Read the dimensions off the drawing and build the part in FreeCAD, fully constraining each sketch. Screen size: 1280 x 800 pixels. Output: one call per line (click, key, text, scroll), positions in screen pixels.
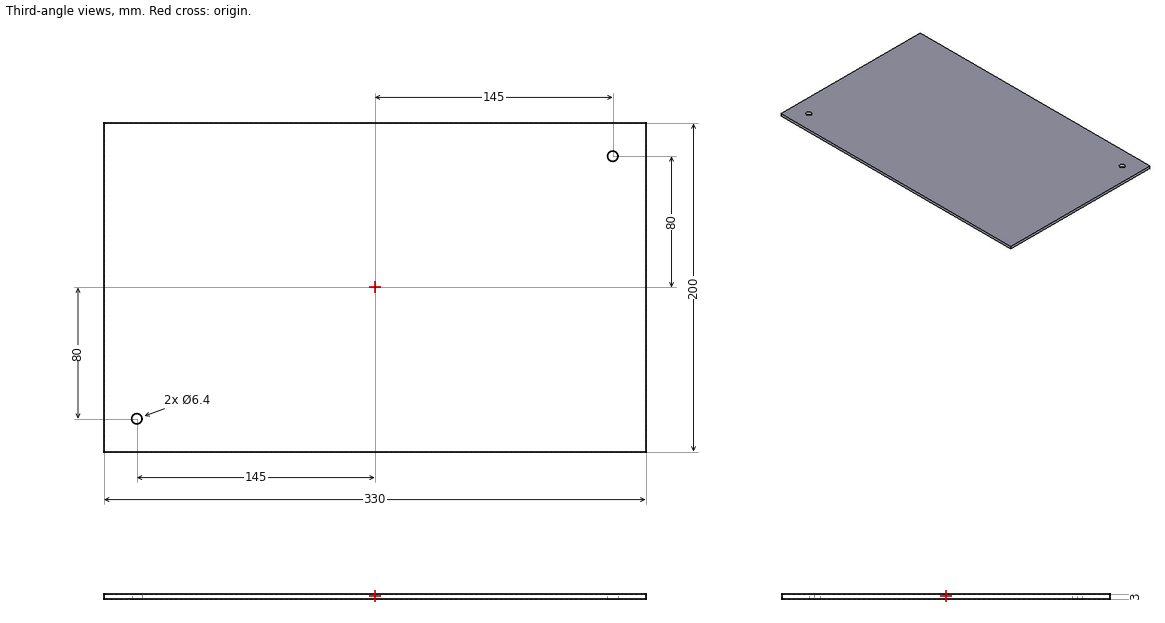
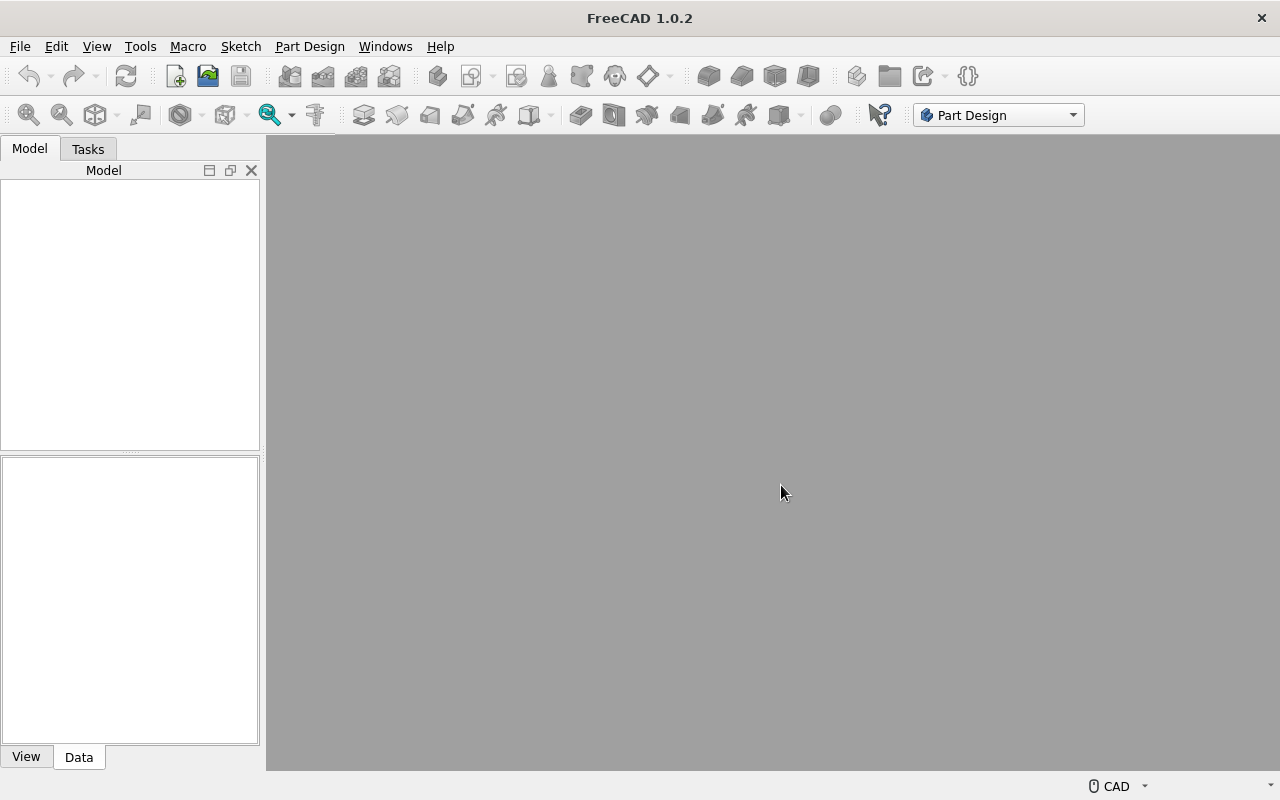
click(175, 76)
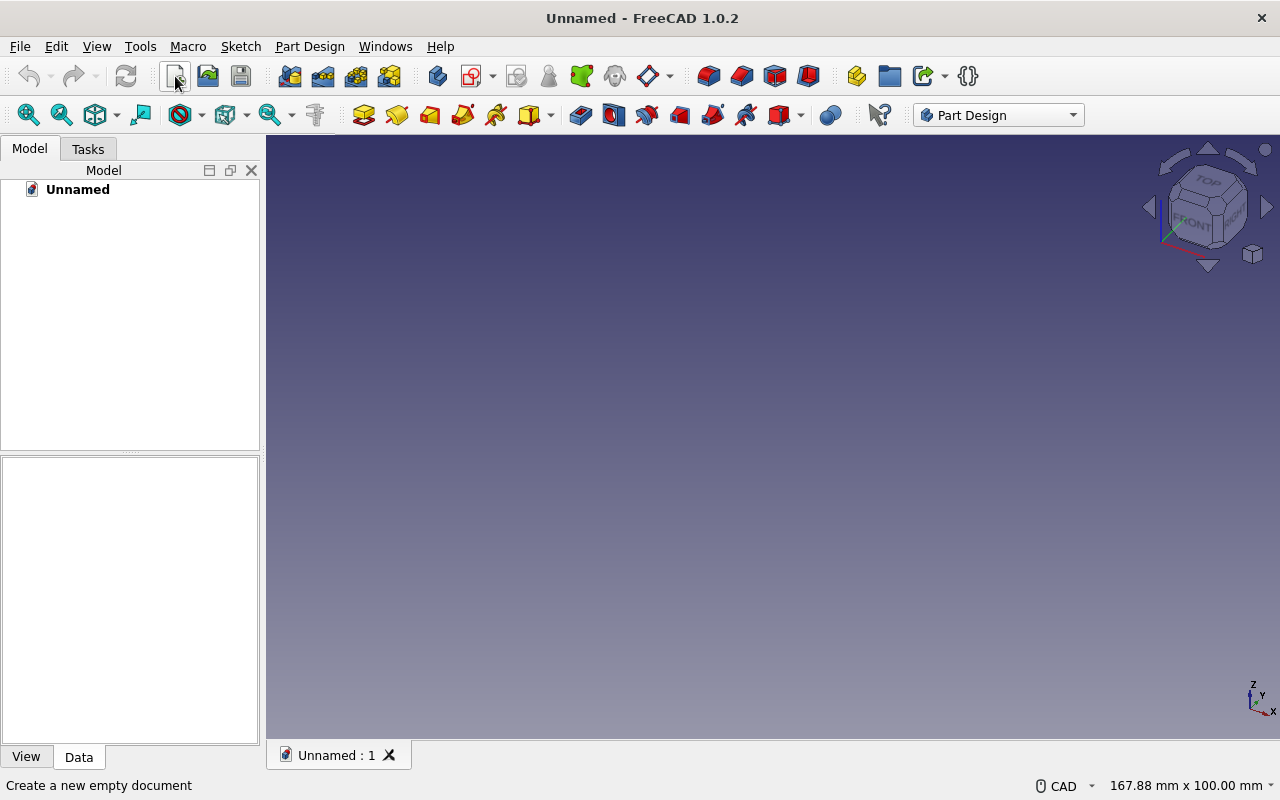
click(470, 76)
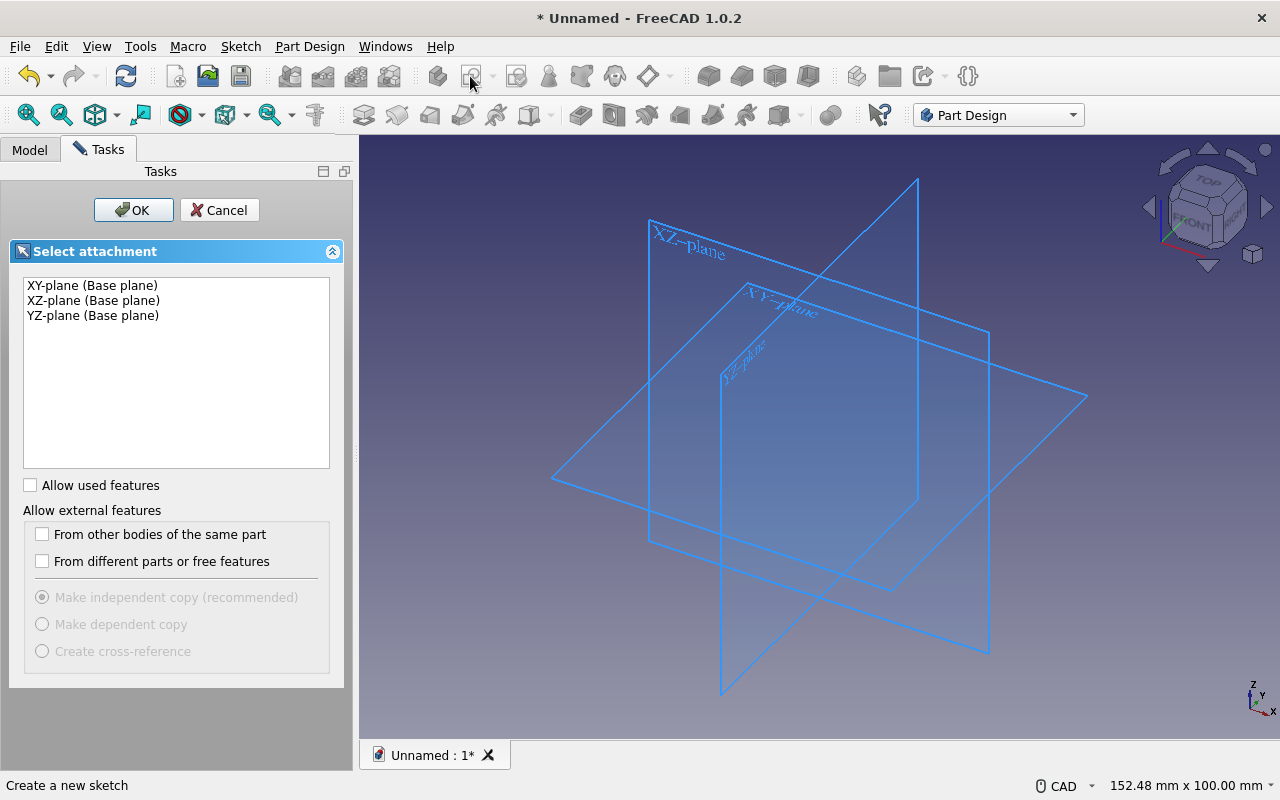
click(84, 286)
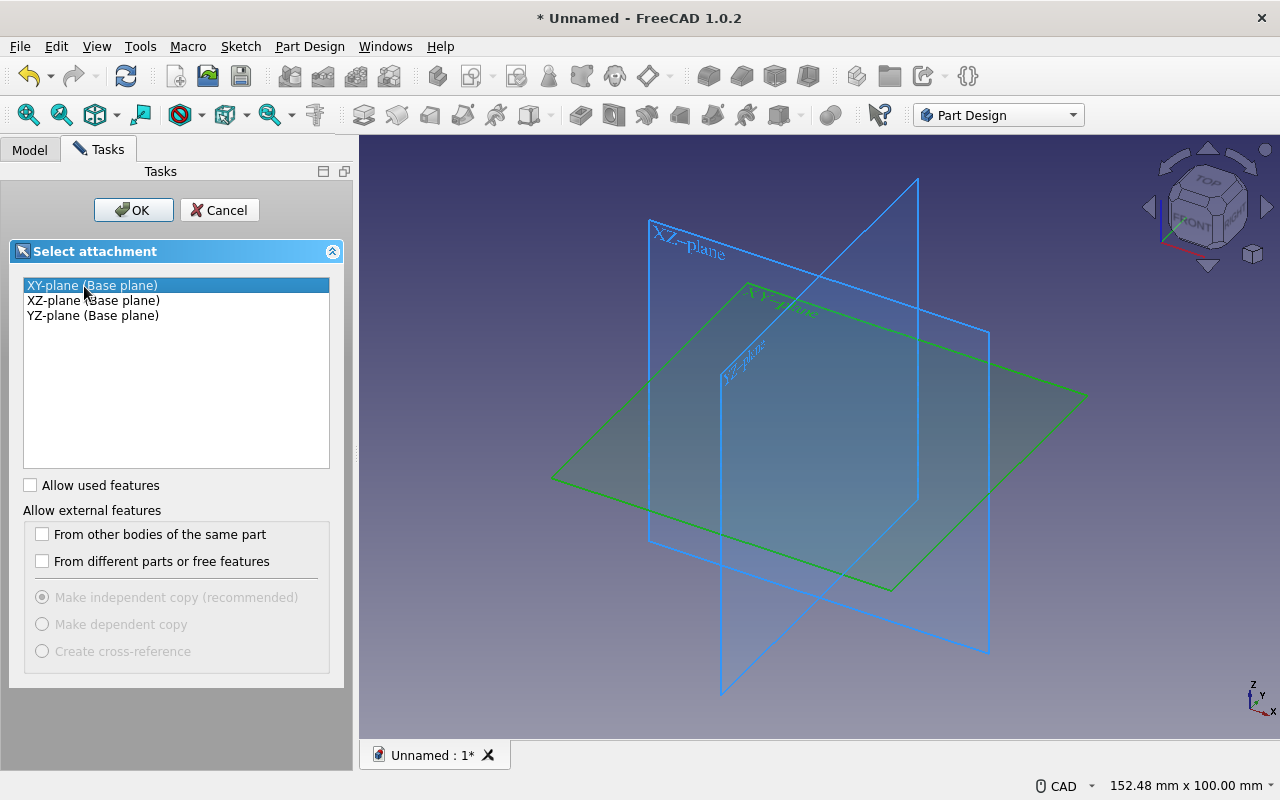
click(134, 210)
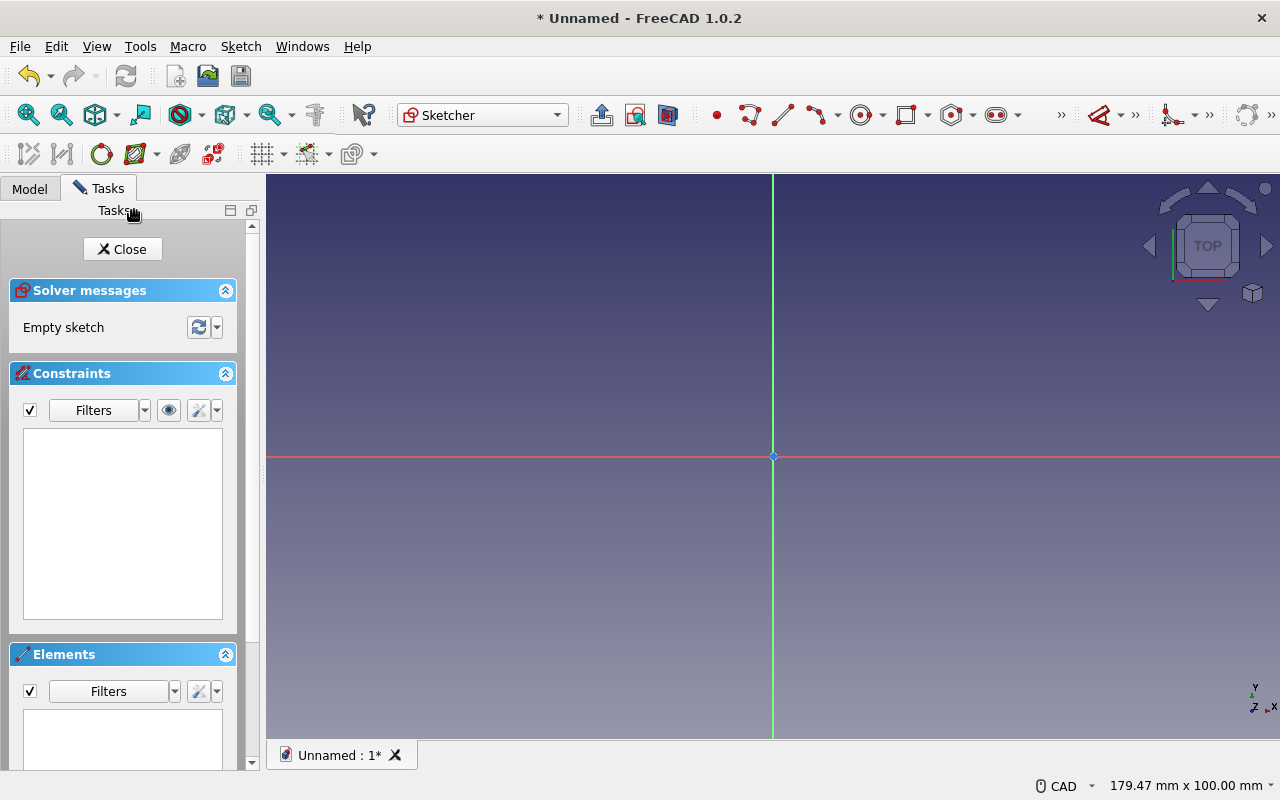
scroll(675, 456, down, 6)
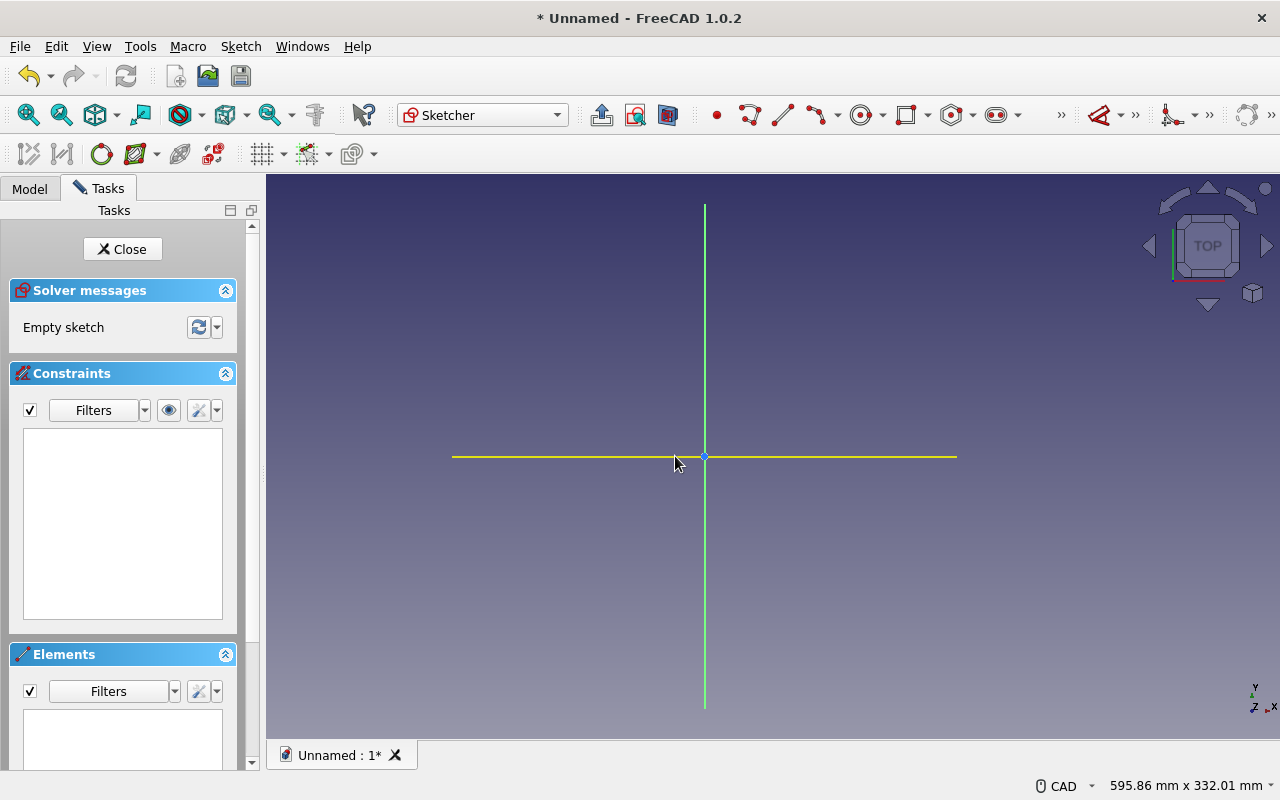
click(928, 116)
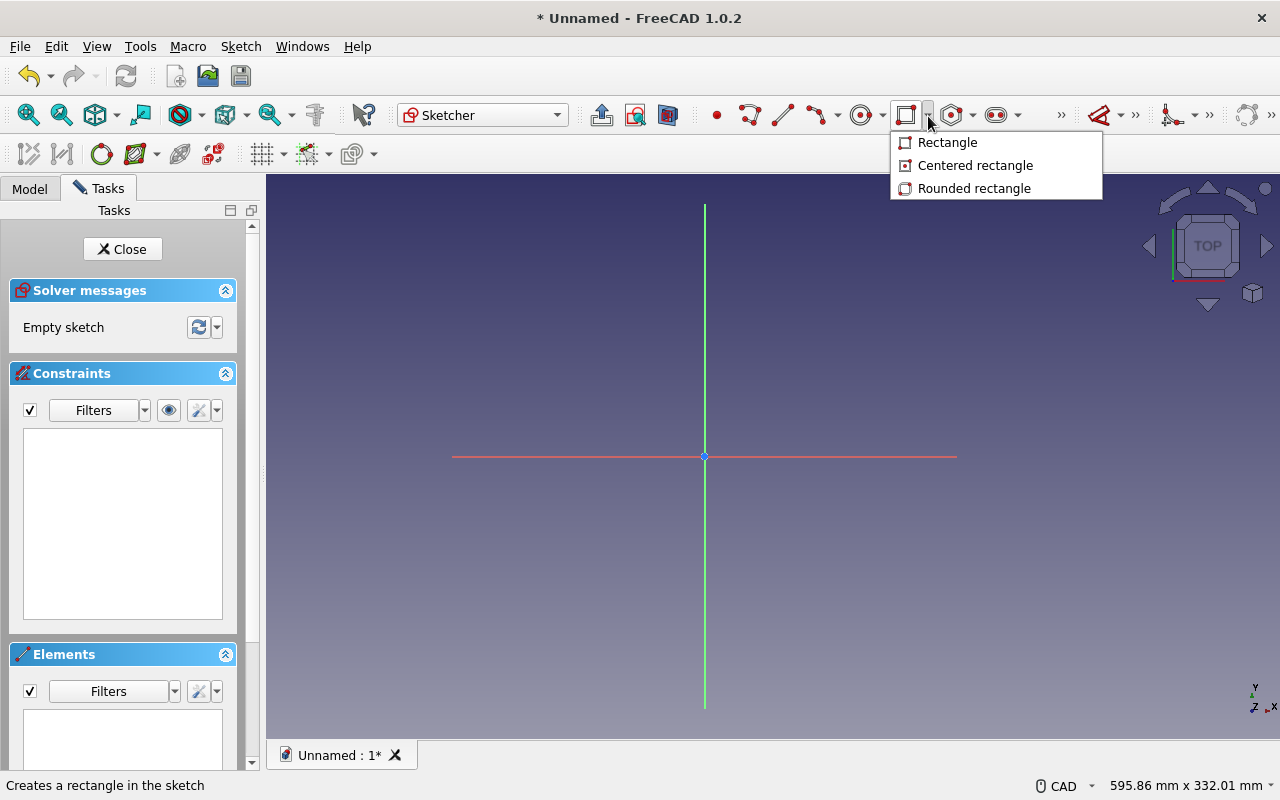
click(996, 166)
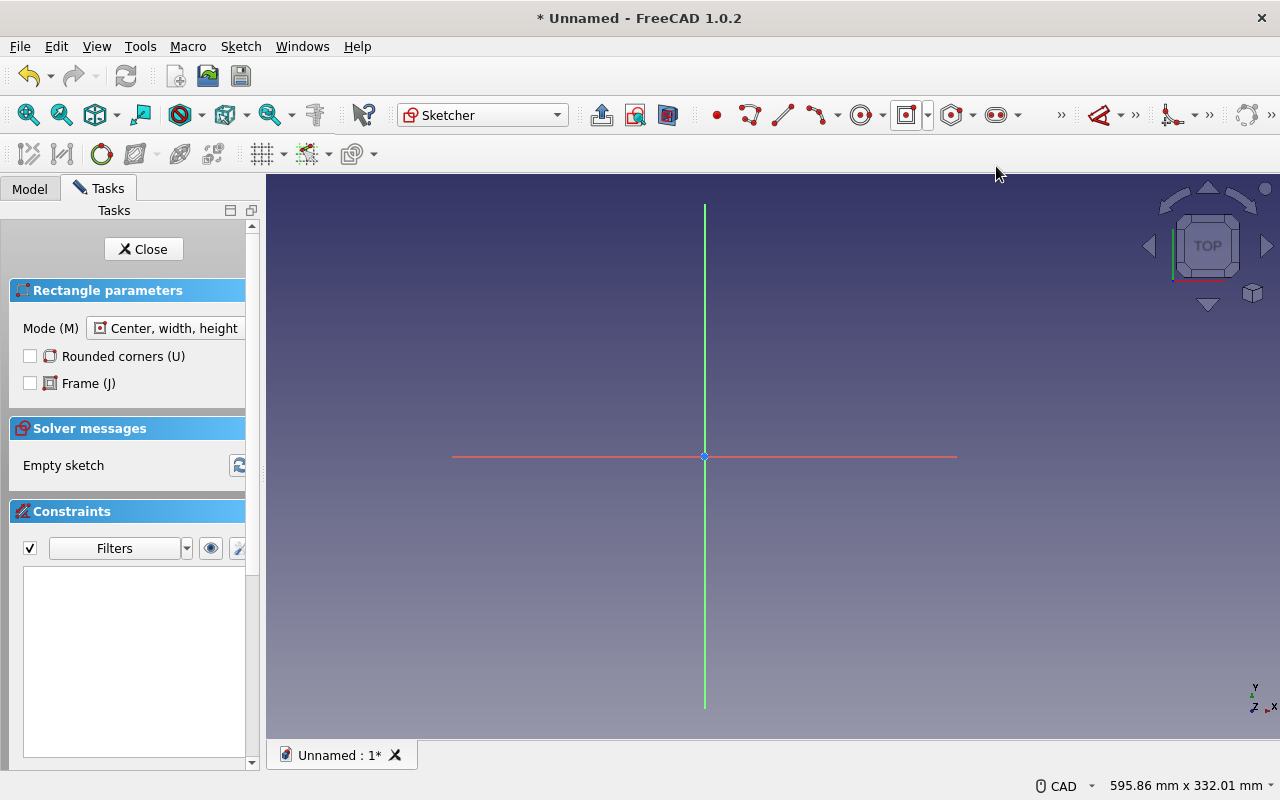
click(705, 456)
move(986, 286)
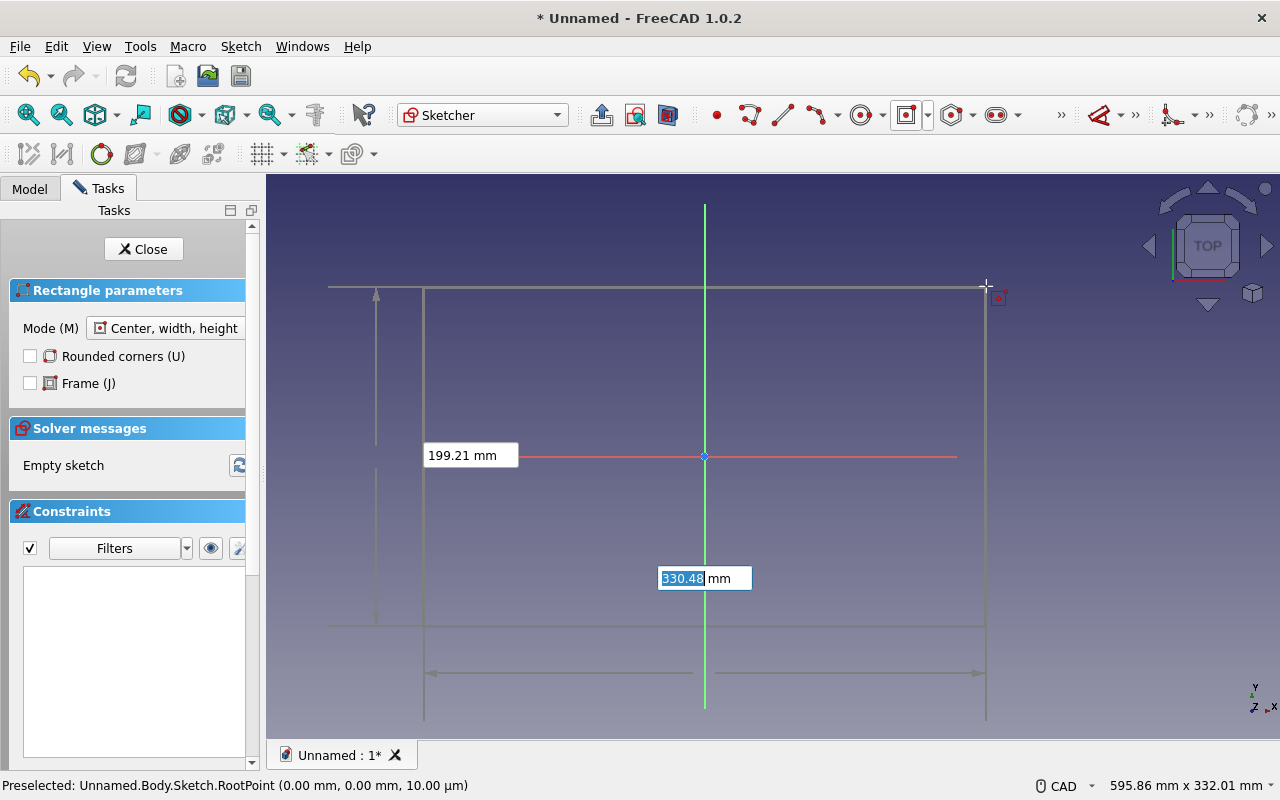
text(330)
key(Tab)
text(200)
key(Return)
key(Escape)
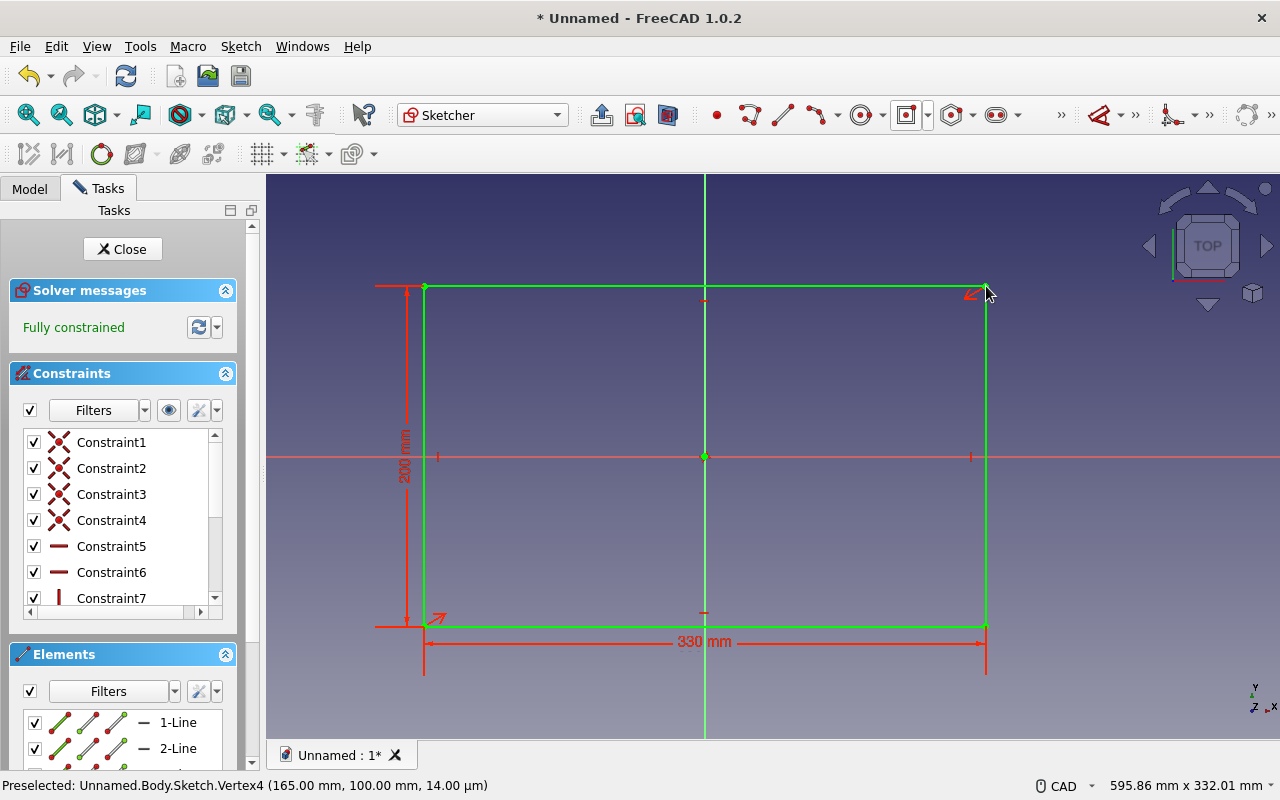
click(123, 249)